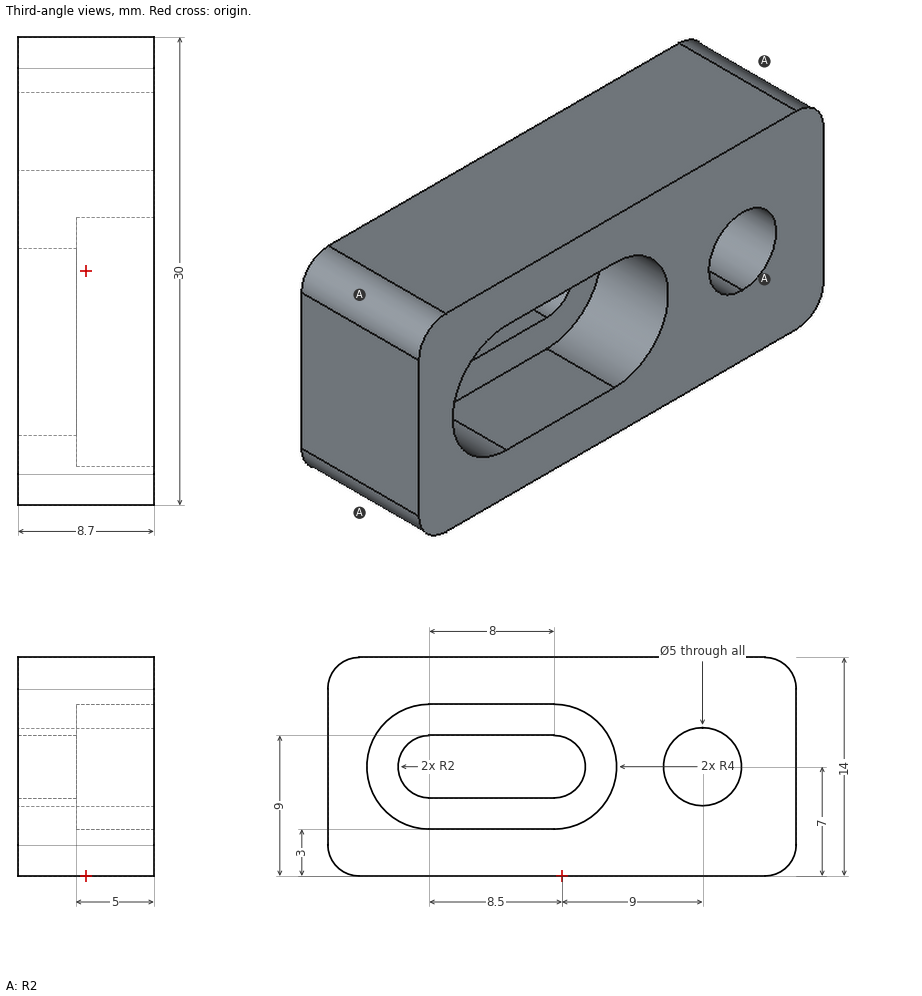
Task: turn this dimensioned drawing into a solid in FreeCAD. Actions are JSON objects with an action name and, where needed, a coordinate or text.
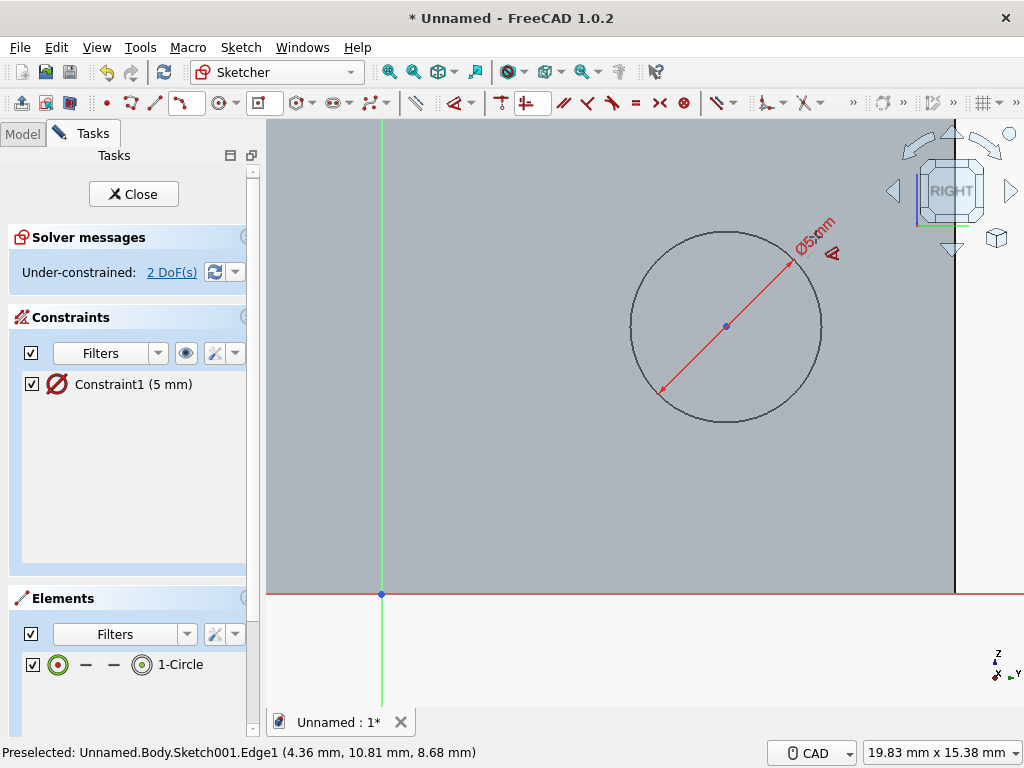
{"action": "left_click", "coordinate": [726, 327]}
{"action": "left_click", "coordinate": [554, 628]}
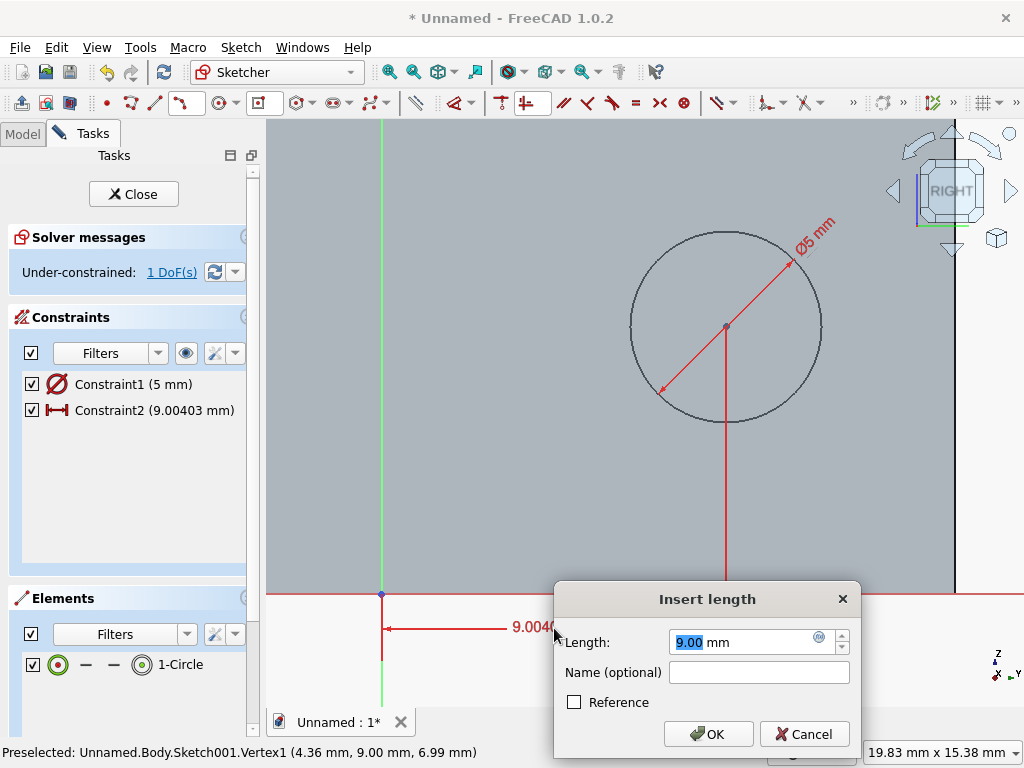
{"action": "type", "text": "9"}
{"action": "key", "text": "Return"}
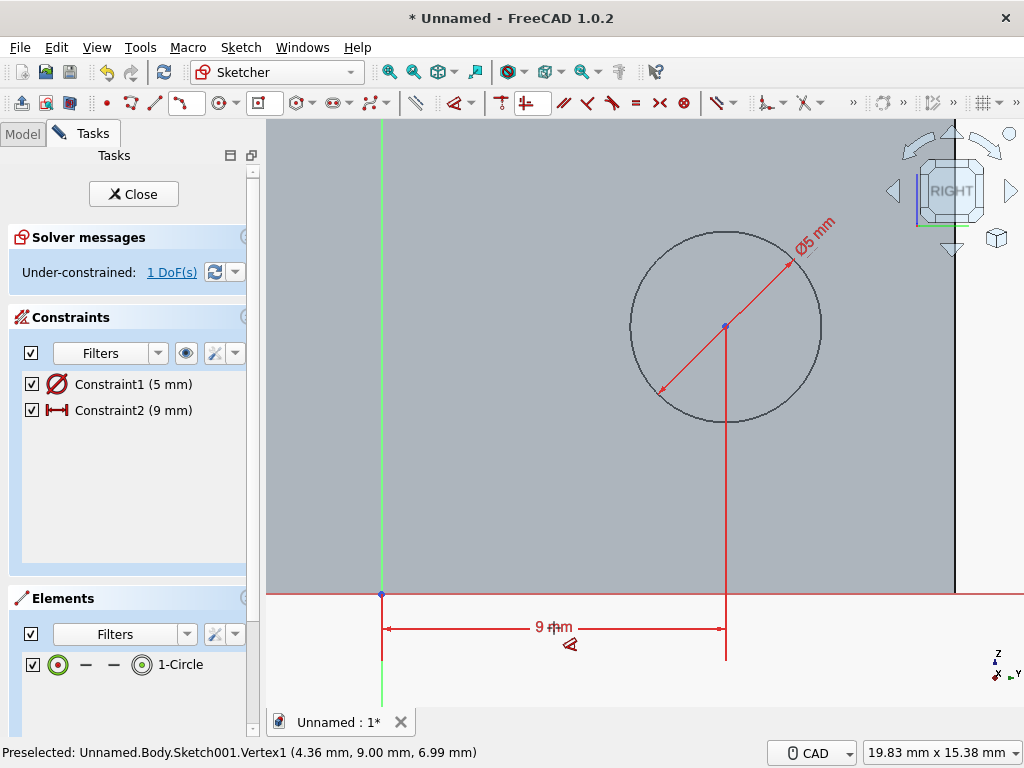
{"action": "left_click", "coordinate": [726, 327]}
{"action": "left_click", "coordinate": [348, 461]}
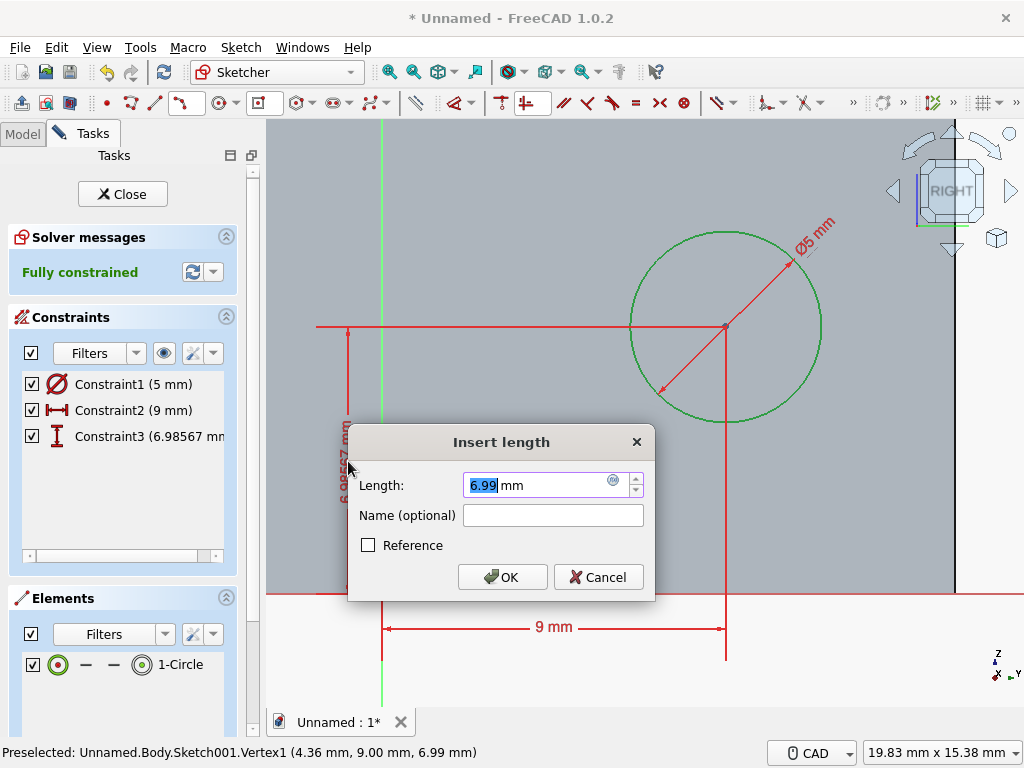
{"action": "type", "text": "7"}
{"action": "key", "text": "Return"}
{"action": "key", "text": "Escape"}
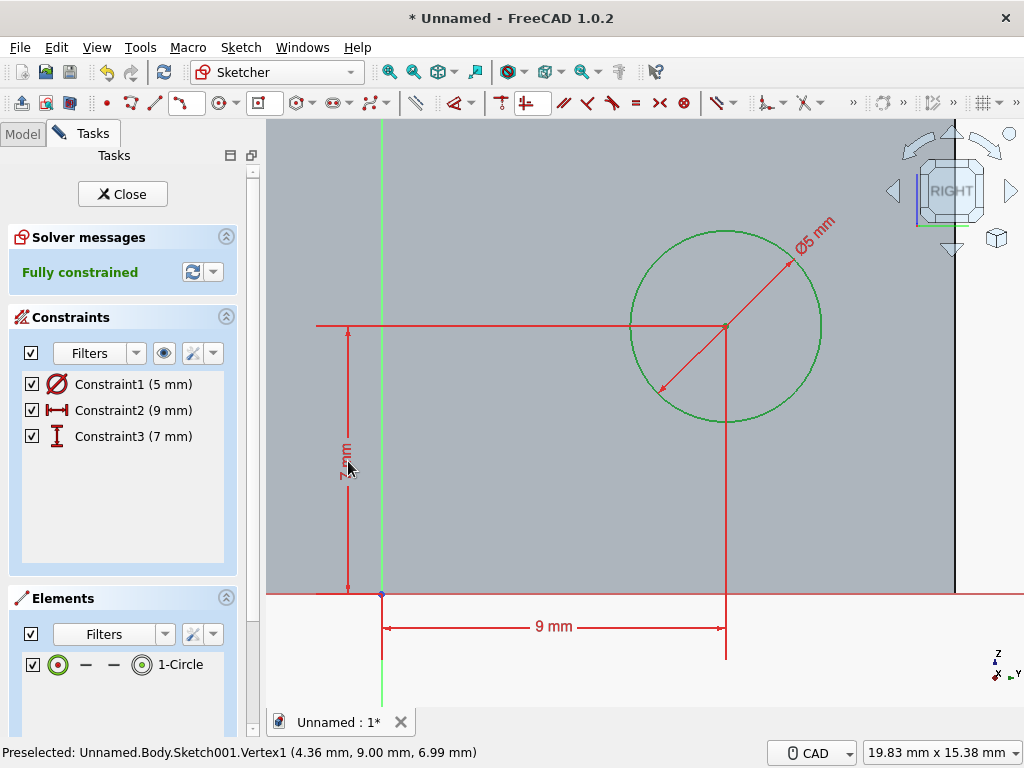
{"action": "left_click", "coordinate": [123, 194]}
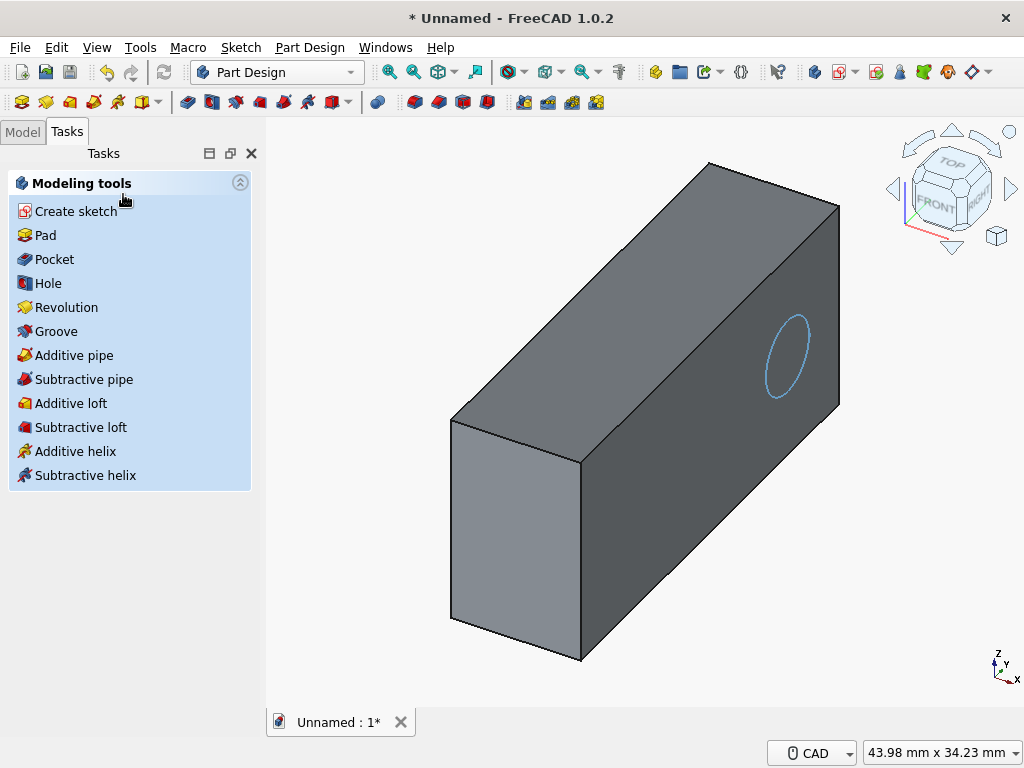
{"action": "left_click", "coordinate": [212, 102]}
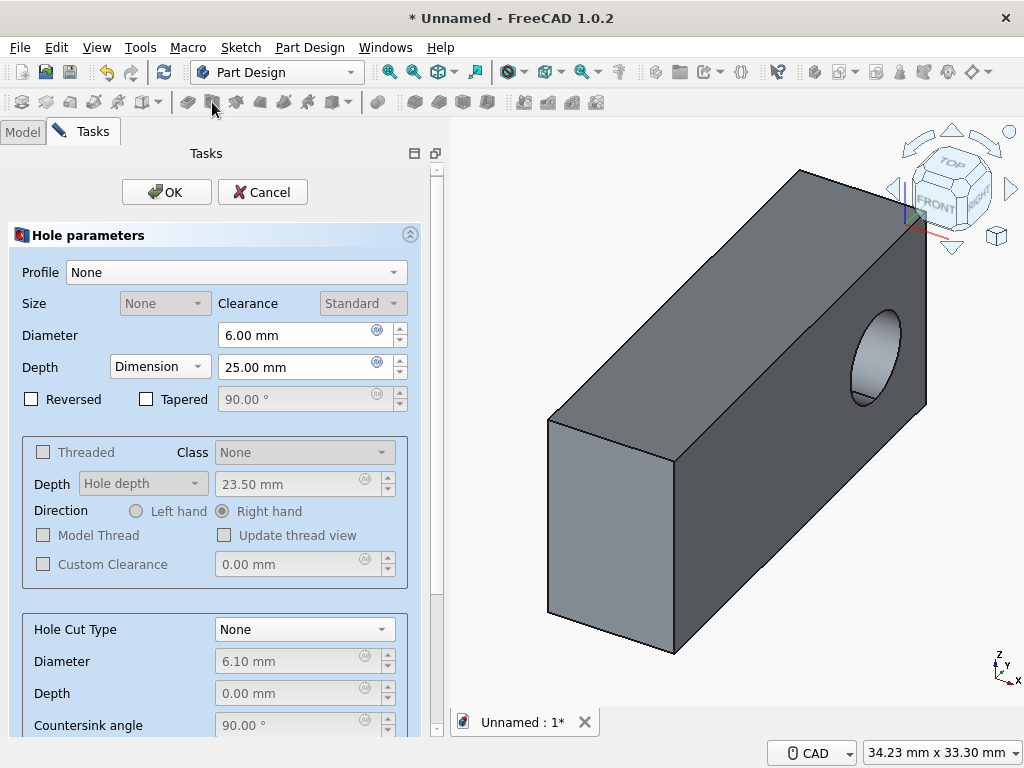
{"action": "triple_click", "coordinate": [305, 335]}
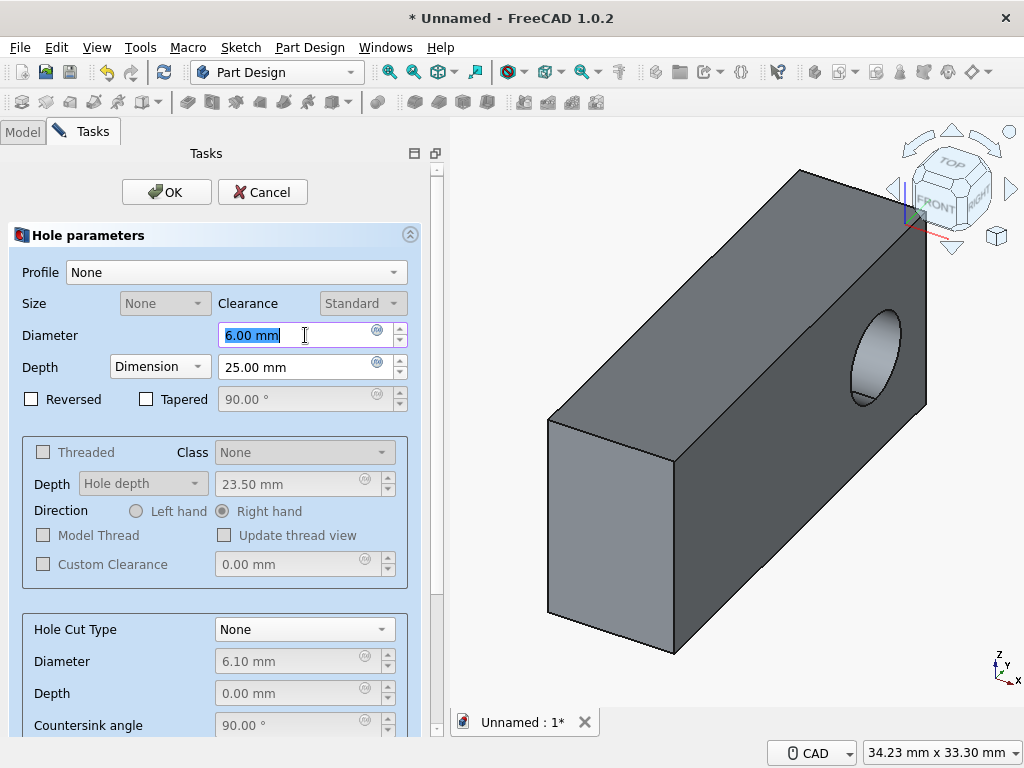
{"action": "type", "text": "5"}
{"action": "key", "text": "Tab"}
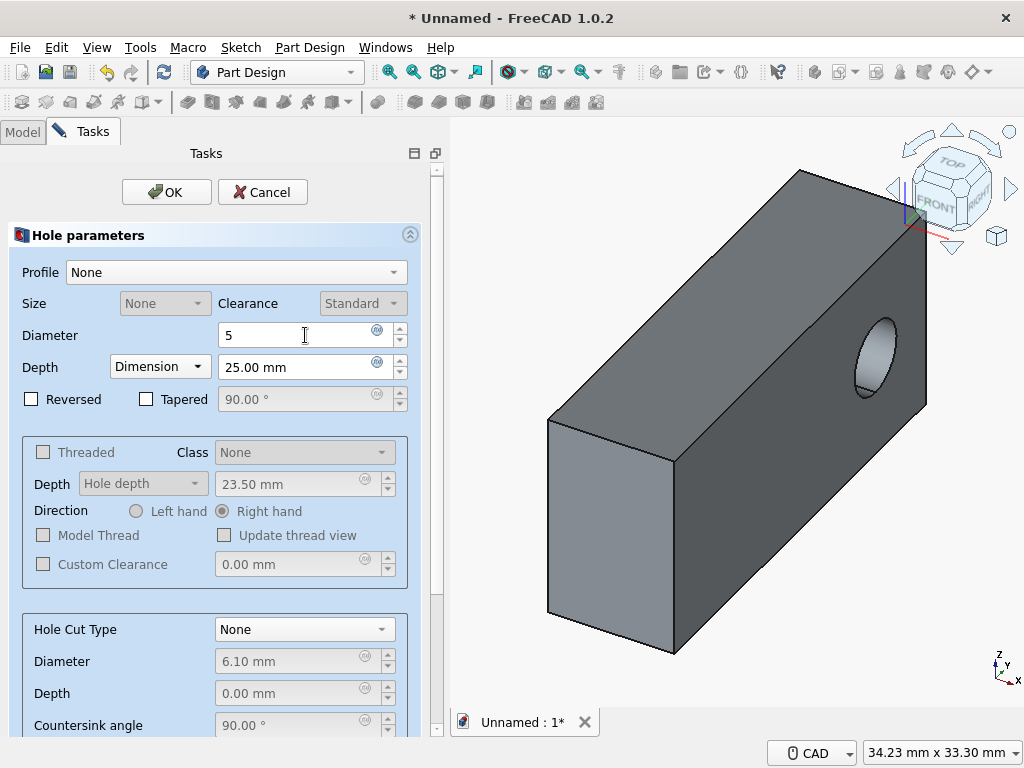
{"action": "left_click", "coordinate": [161, 366]}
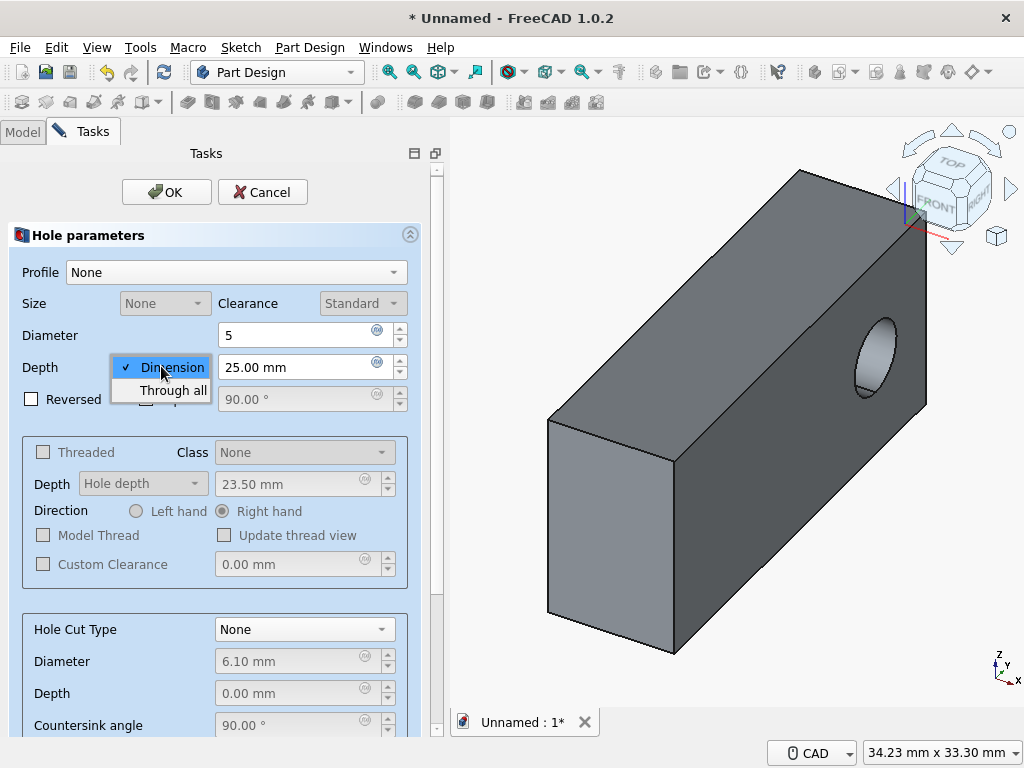
{"action": "left_click", "coordinate": [160, 390]}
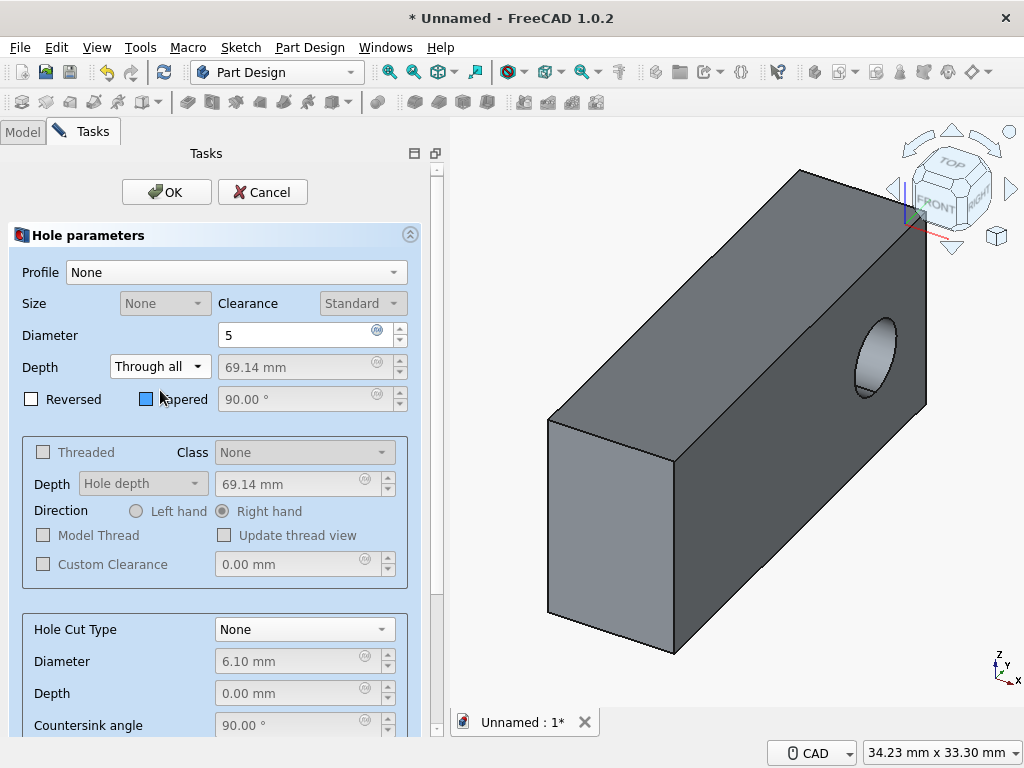
{"action": "left_click", "coordinate": [167, 192]}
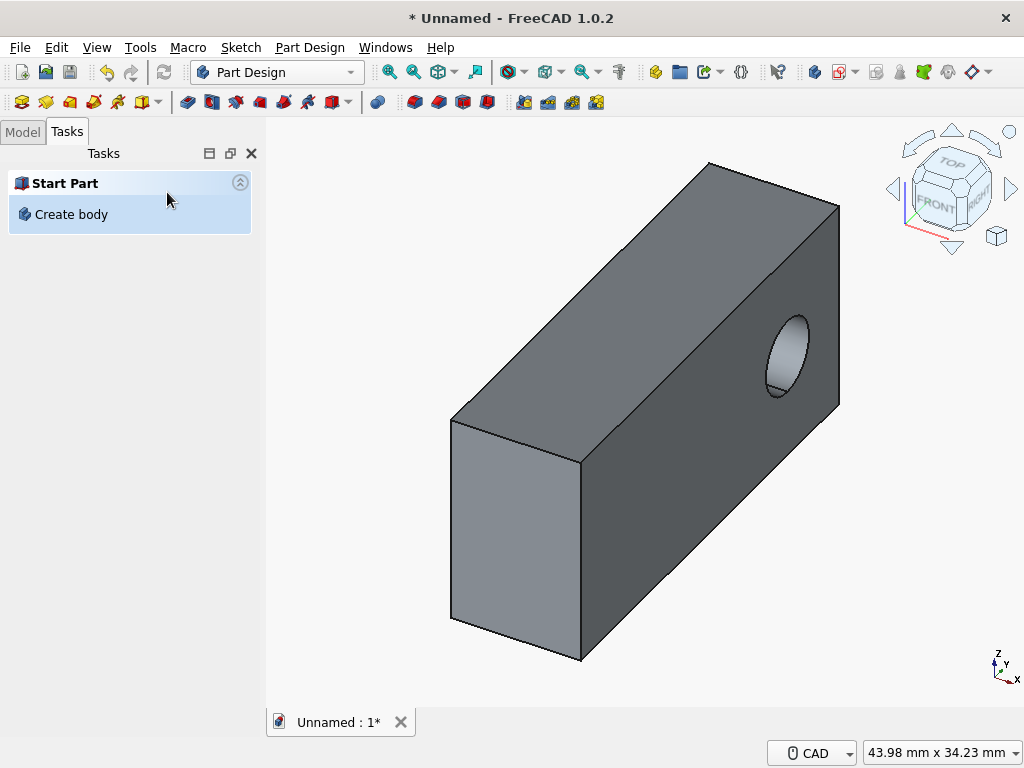
{"action": "left_click", "coordinate": [673, 469]}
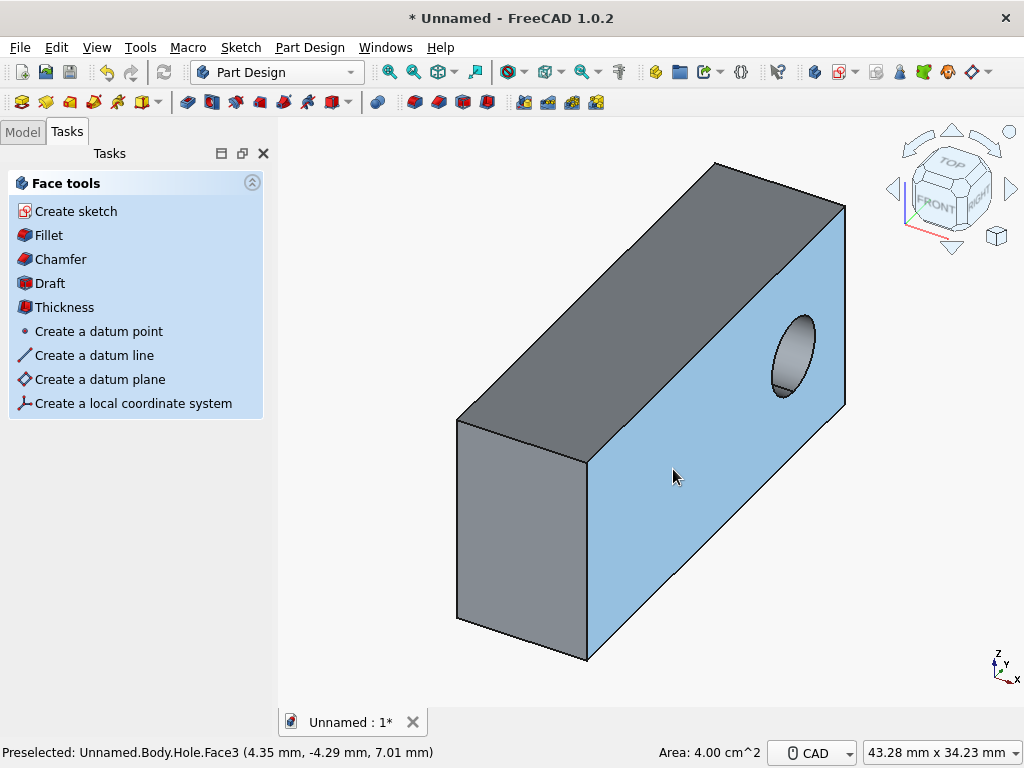
{"action": "left_click", "coordinate": [840, 72]}